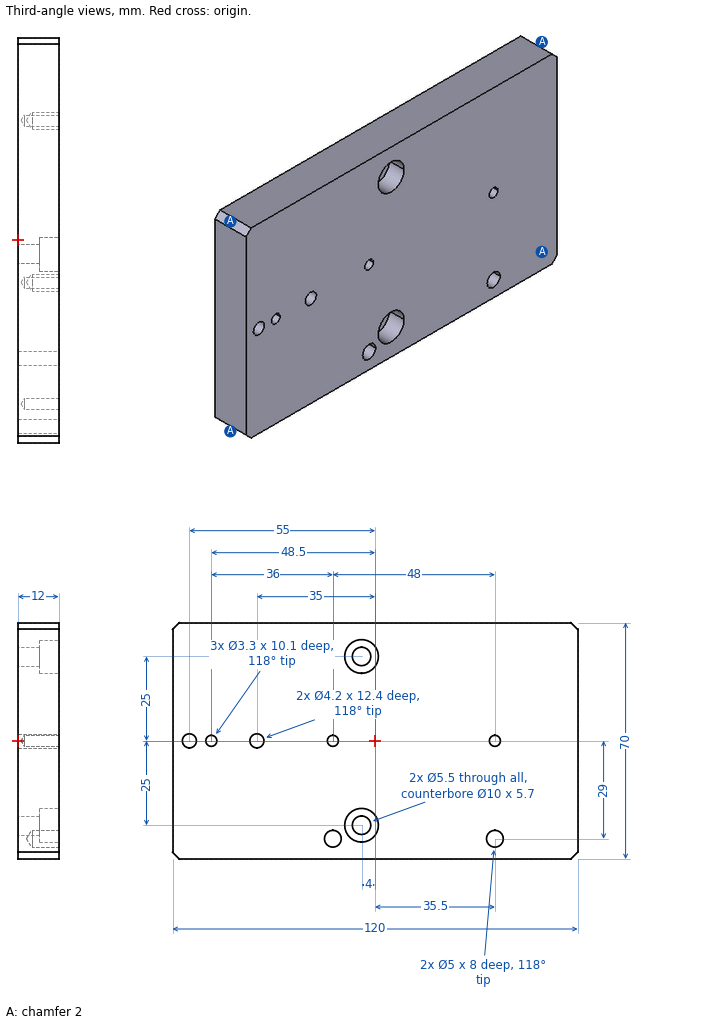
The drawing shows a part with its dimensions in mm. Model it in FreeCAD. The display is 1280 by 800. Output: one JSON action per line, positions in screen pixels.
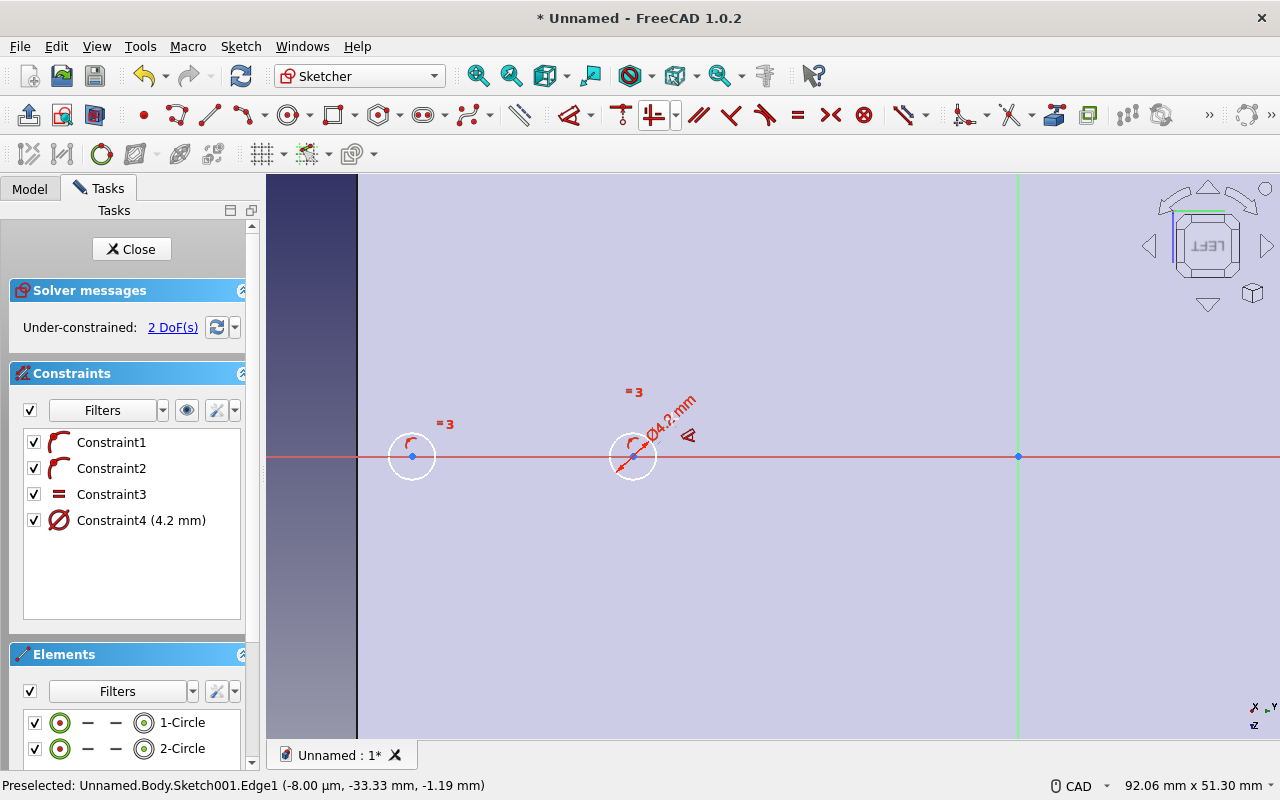
{"action": "left_click", "coordinate": [633, 456]}
{"action": "left_click", "coordinate": [826, 490]}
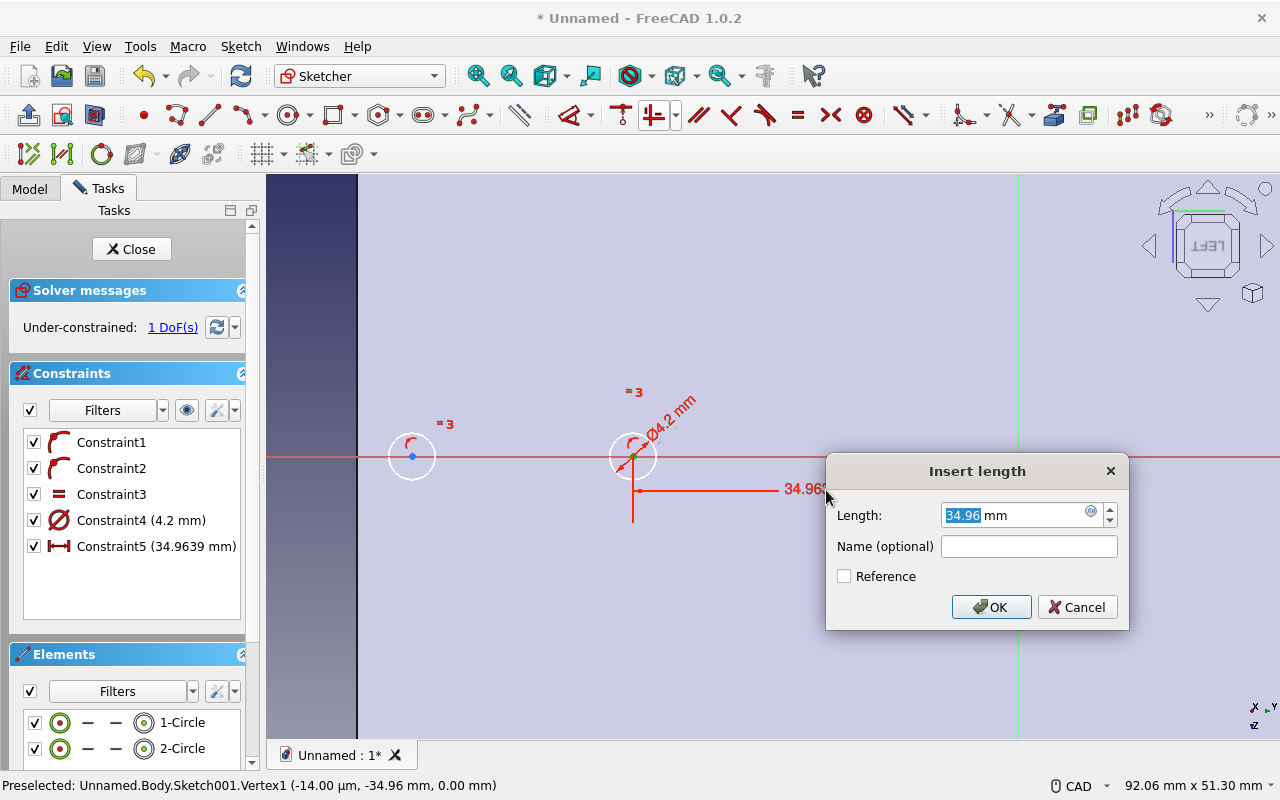
{"action": "type", "text": "35"}
{"action": "key", "text": "Return"}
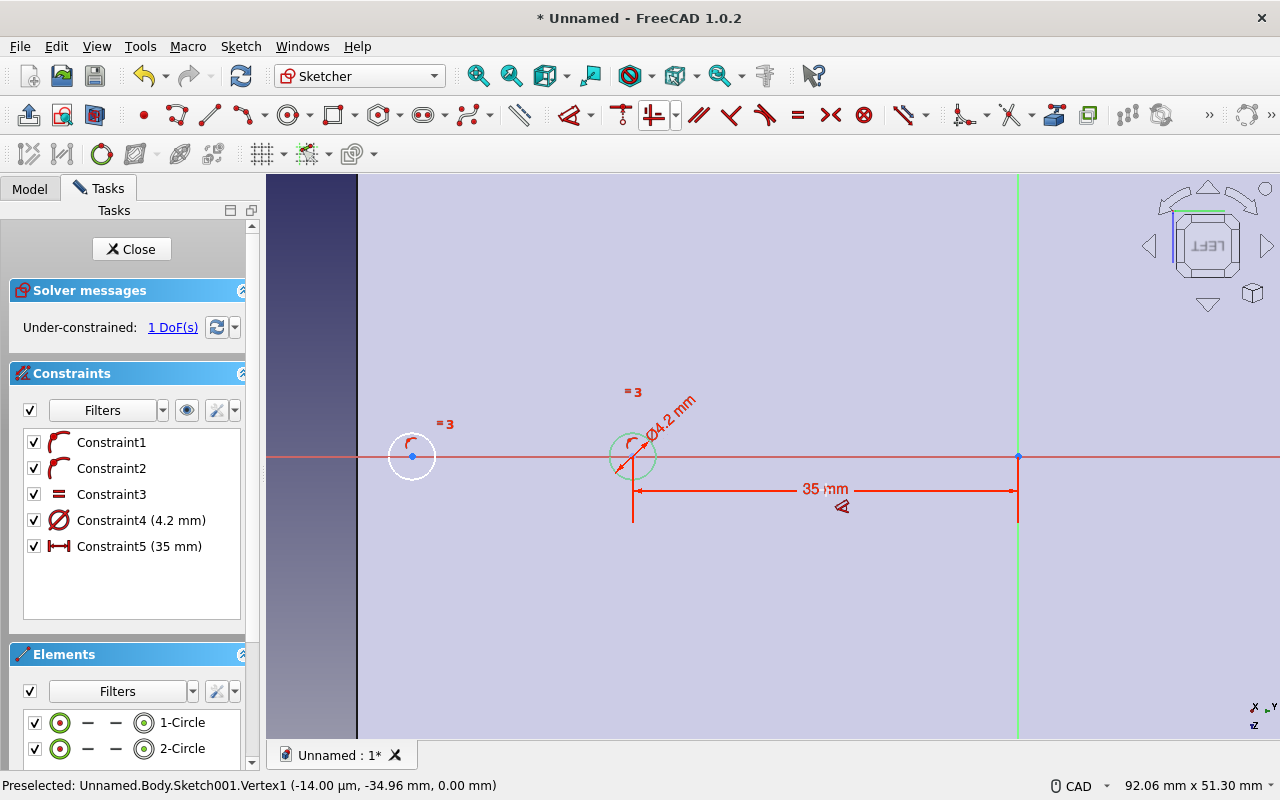
{"action": "left_click", "coordinate": [412, 456]}
{"action": "left_click", "coordinate": [715, 490]}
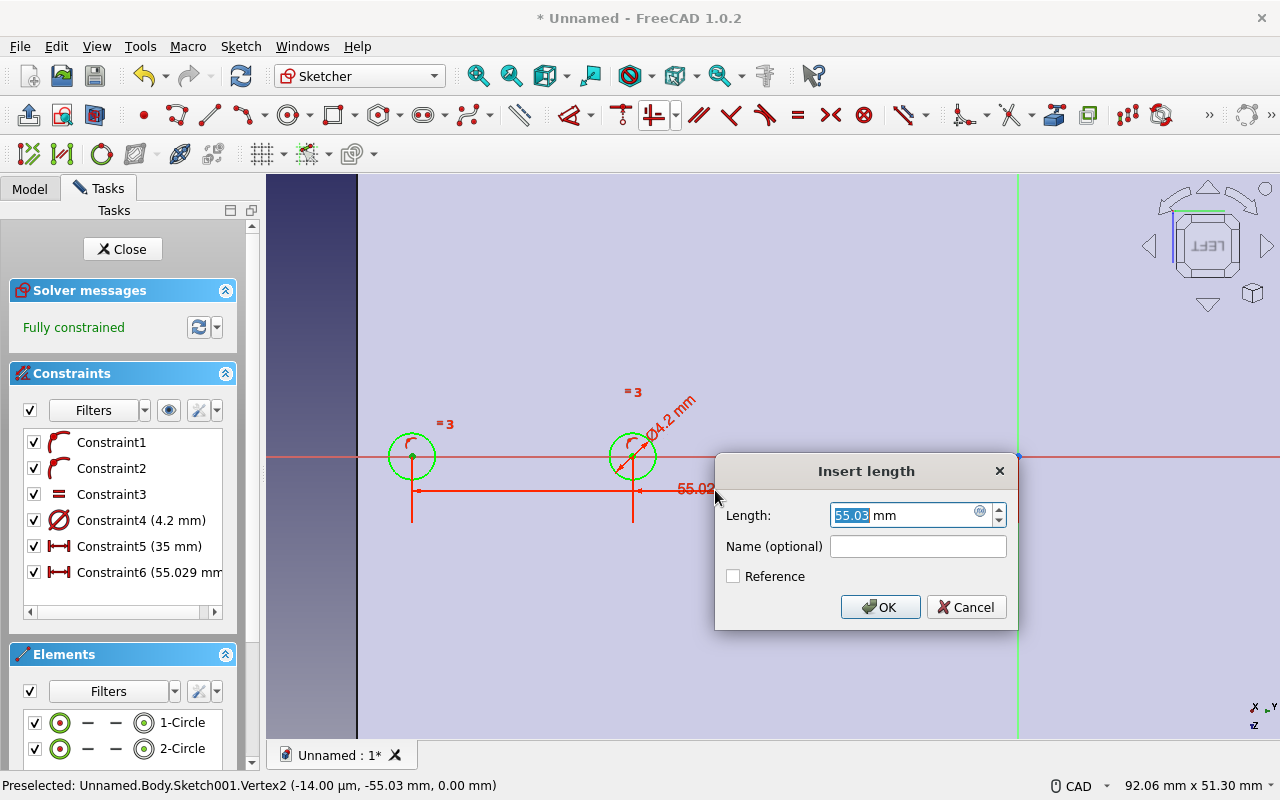
{"action": "type", "text": "55"}
{"action": "key", "text": "Return"}
{"action": "key", "text": "Escape"}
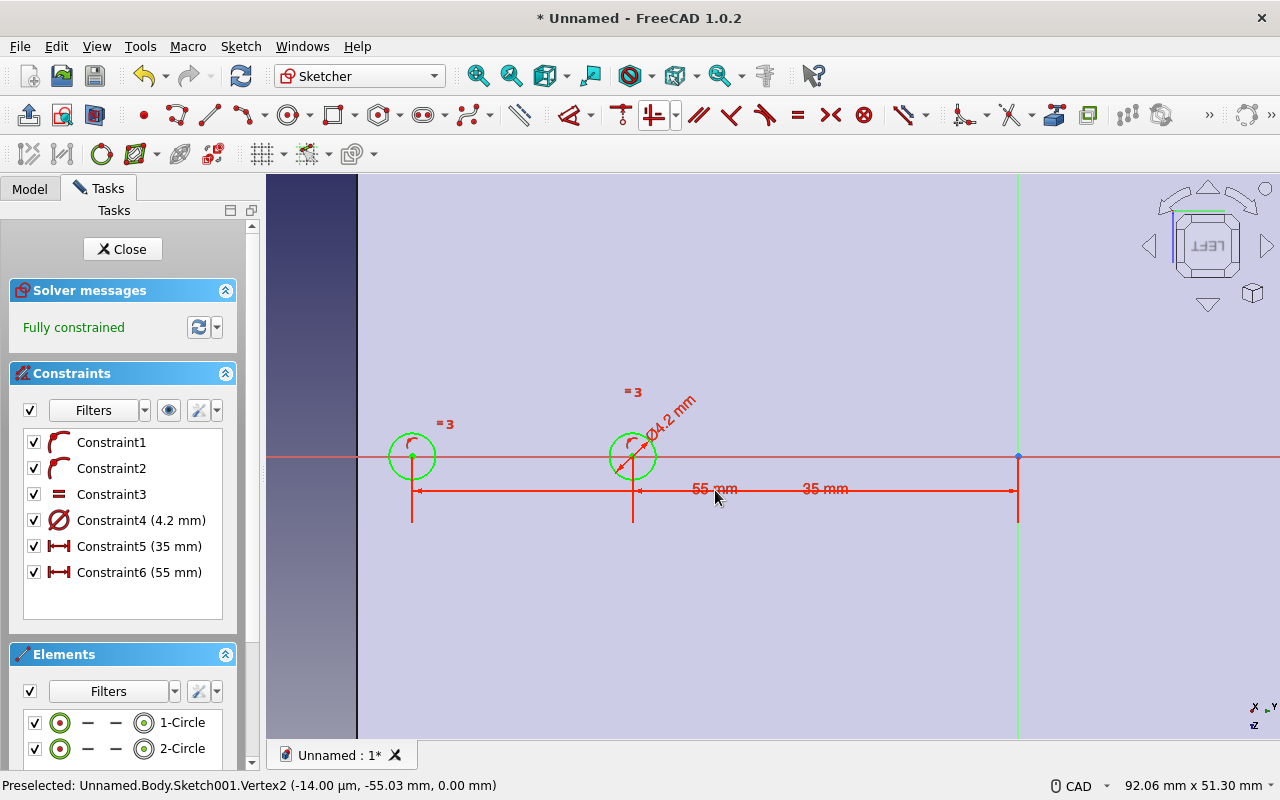
{"action": "left_click", "coordinate": [123, 249]}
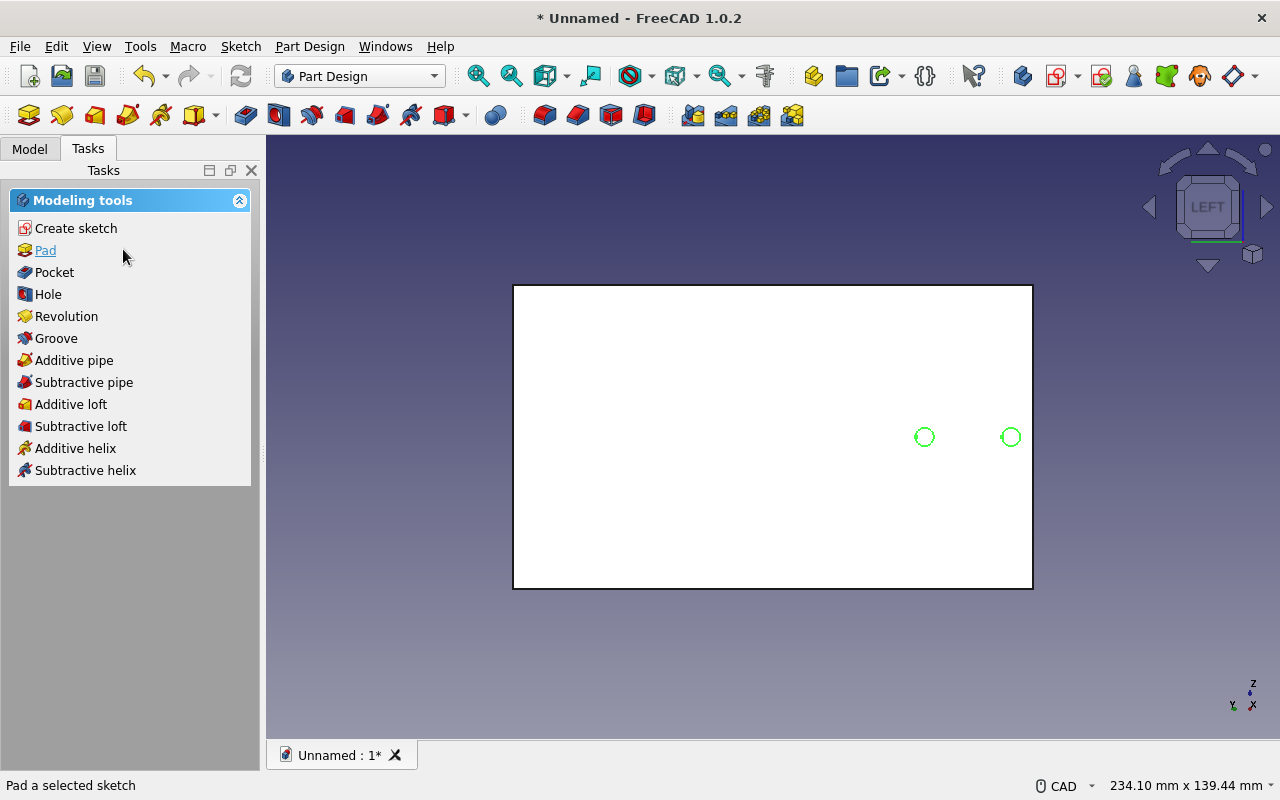
{"action": "left_click", "coordinate": [279, 116]}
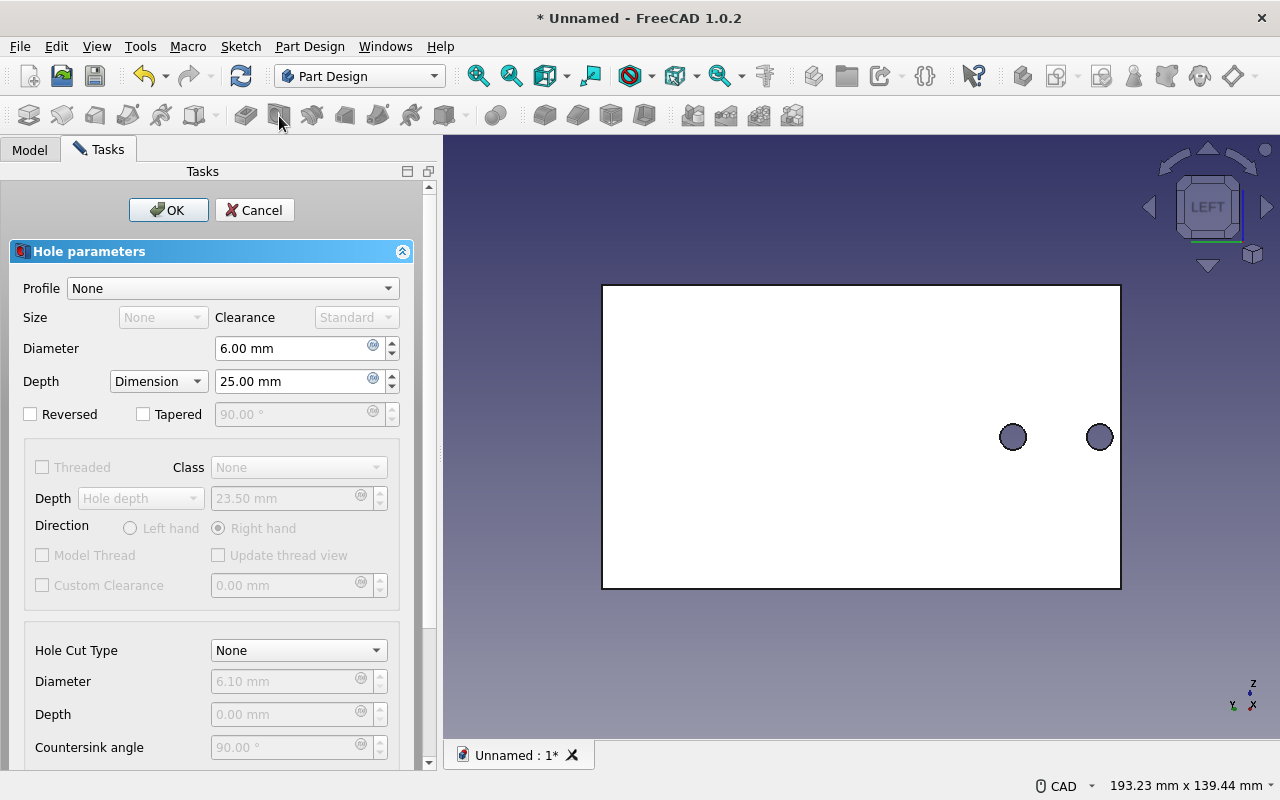
{"action": "triple_click", "coordinate": [300, 348]}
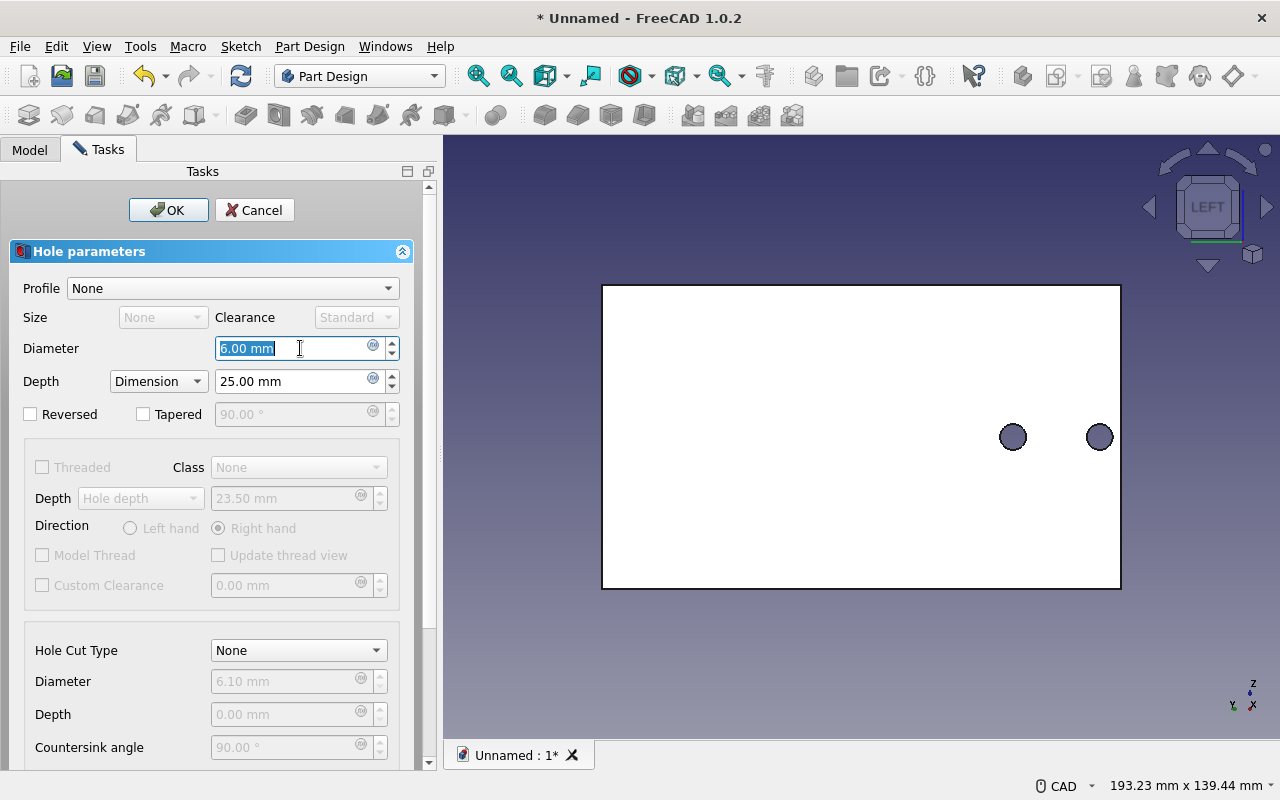
{"action": "type", "text": "4.2"}
{"action": "key", "text": "Tab"}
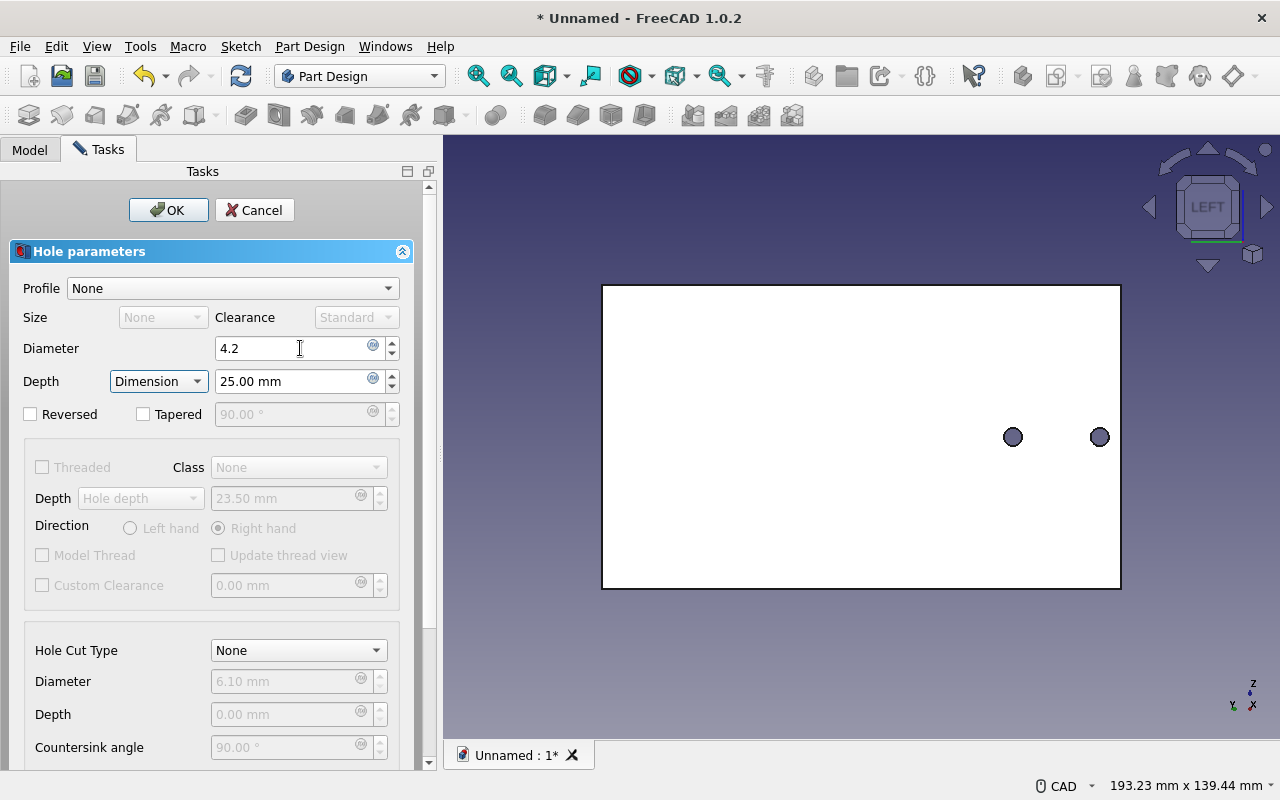
{"action": "triple_click", "coordinate": [300, 382]}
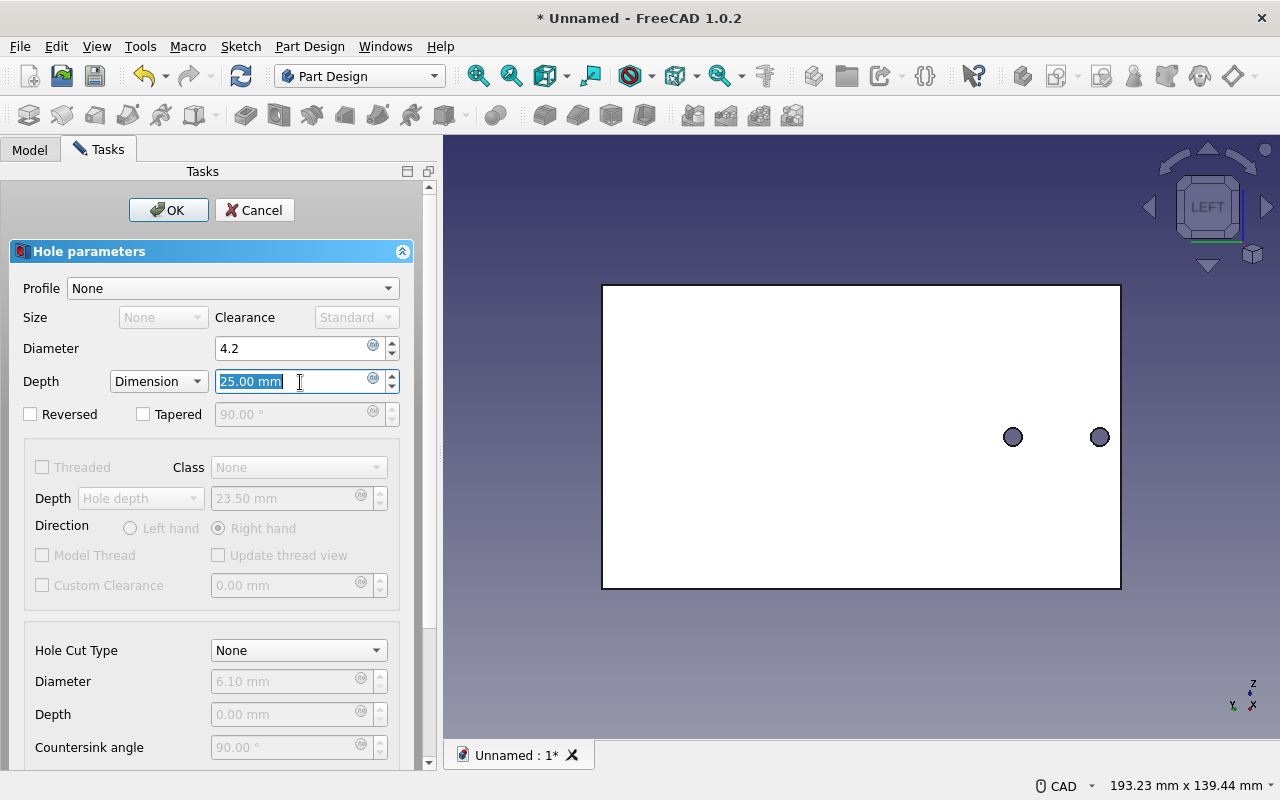
{"action": "type", "text": "12.4"}
{"action": "key", "text": "Tab"}